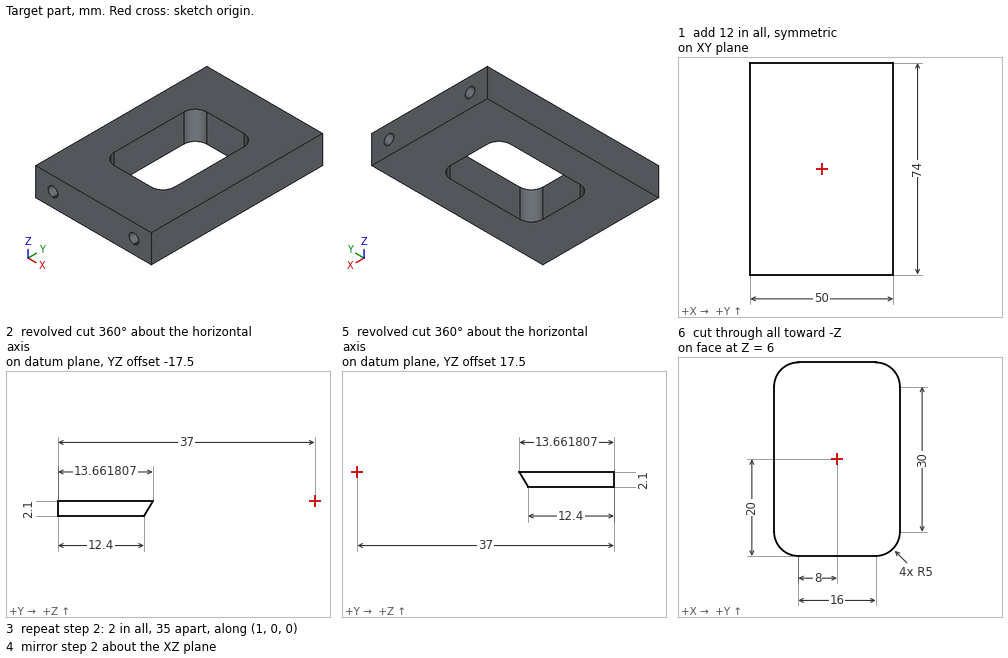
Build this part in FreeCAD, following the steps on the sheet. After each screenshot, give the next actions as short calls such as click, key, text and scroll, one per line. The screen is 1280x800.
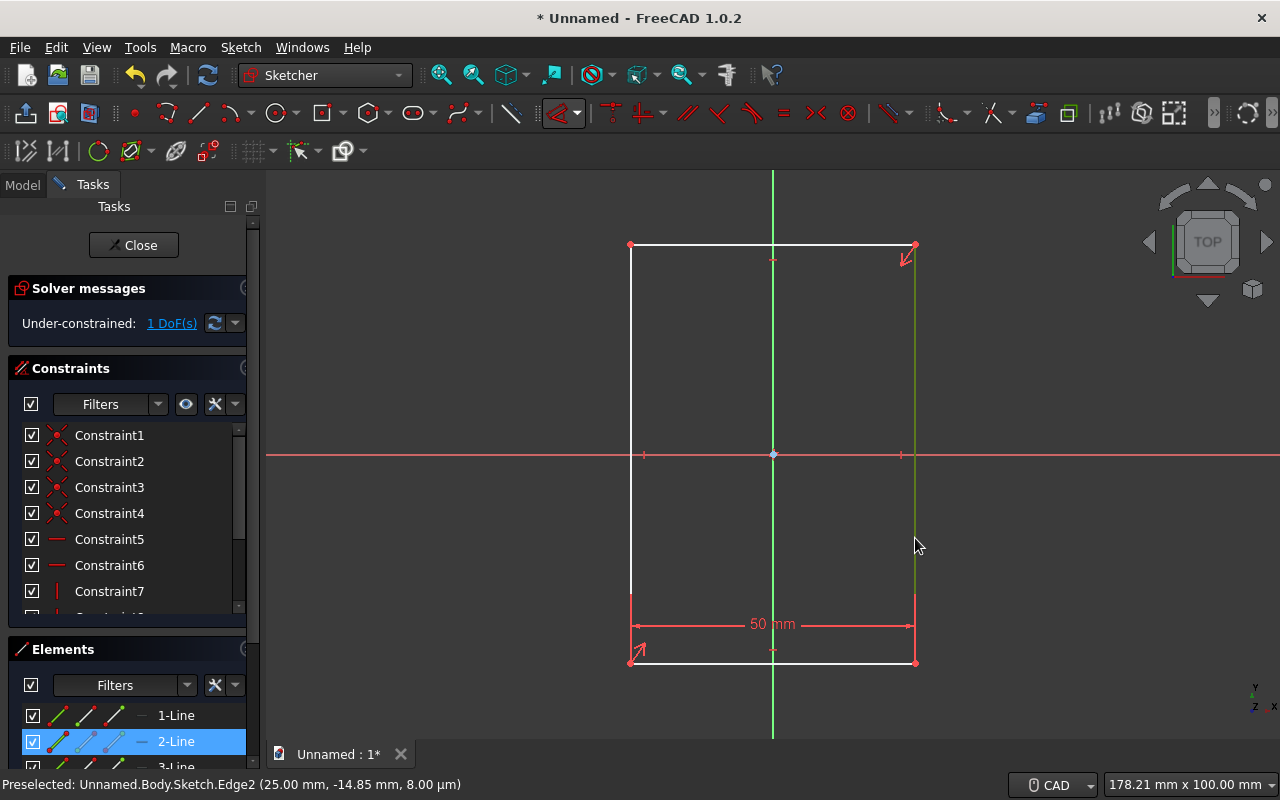
click(580, 114)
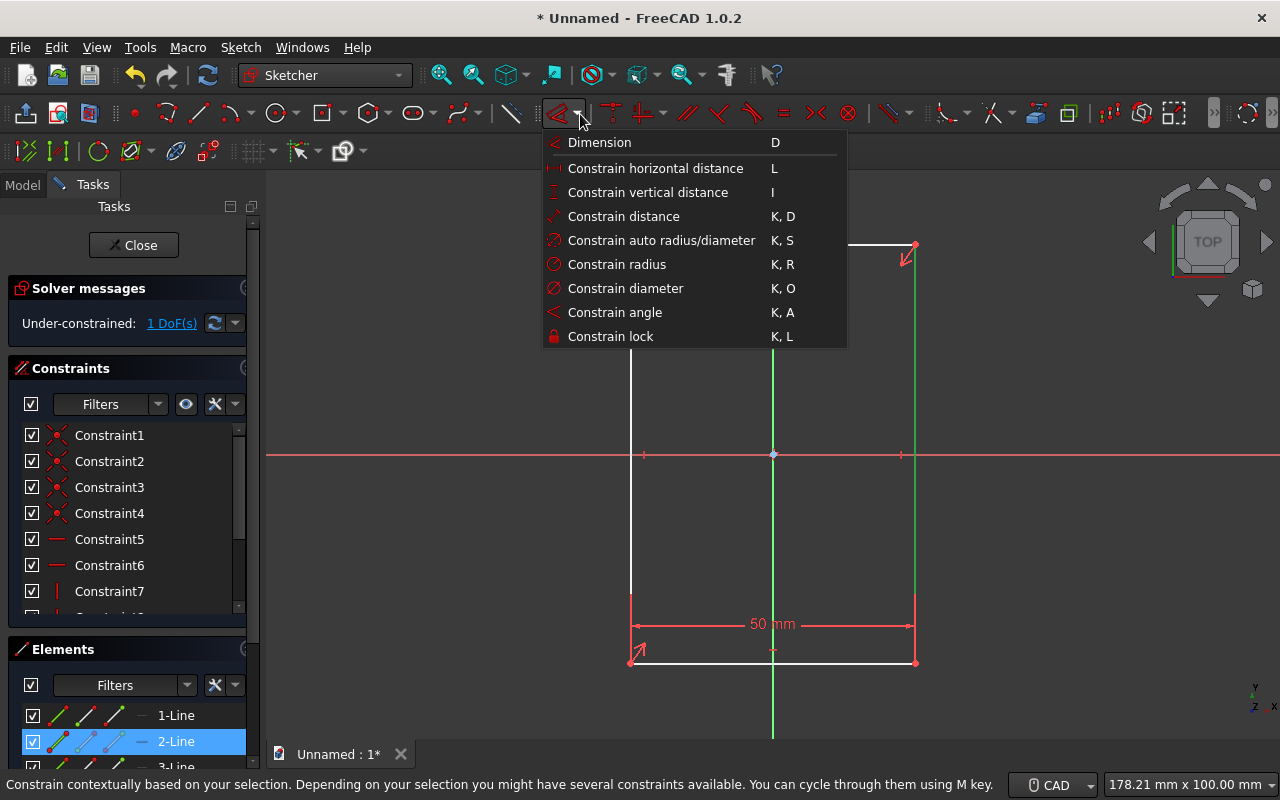
click(695, 192)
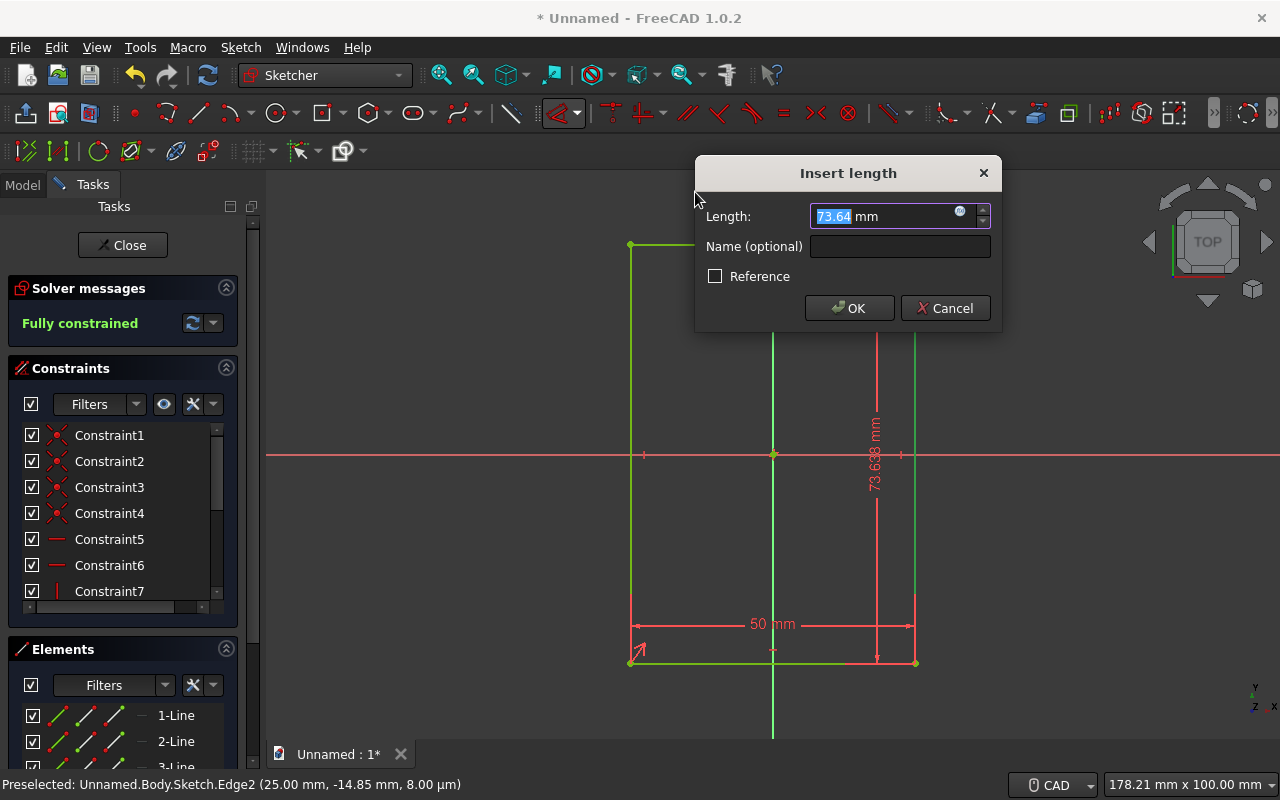
text(74)
key(Return)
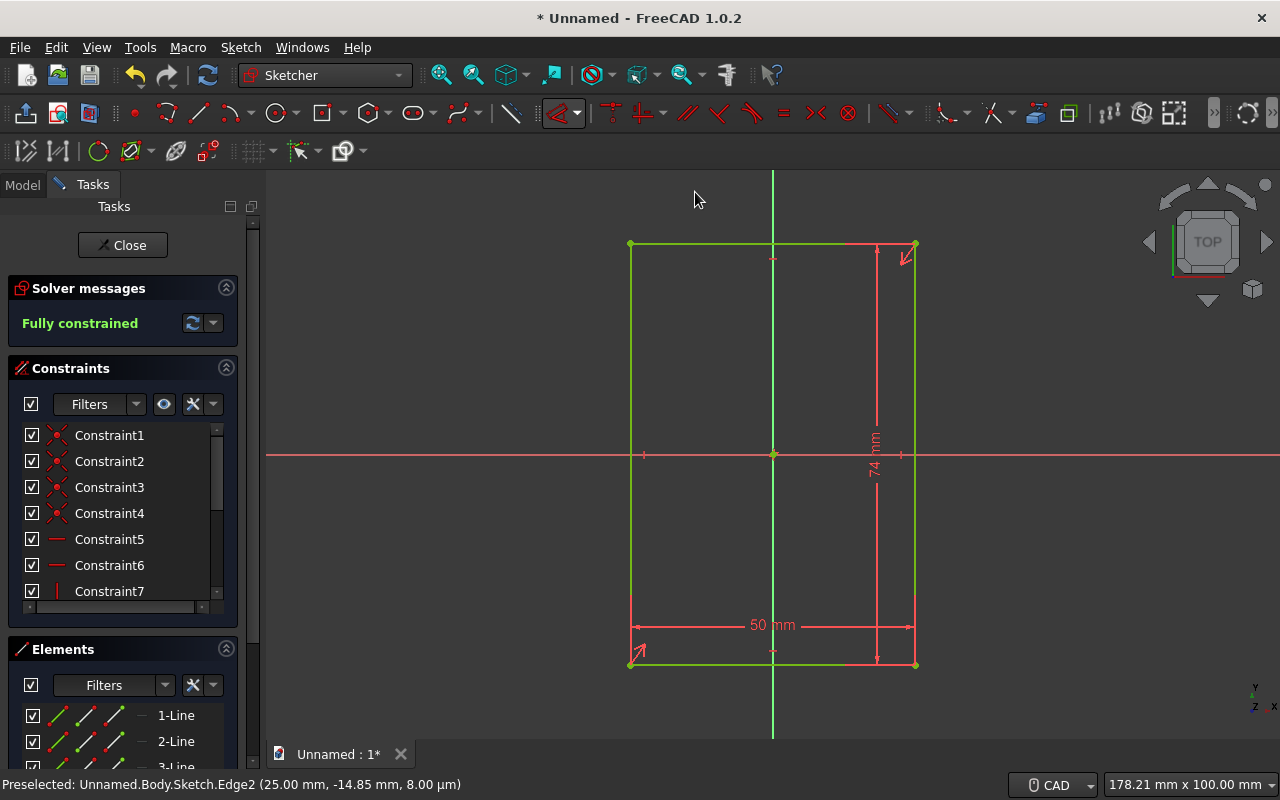
click(123, 245)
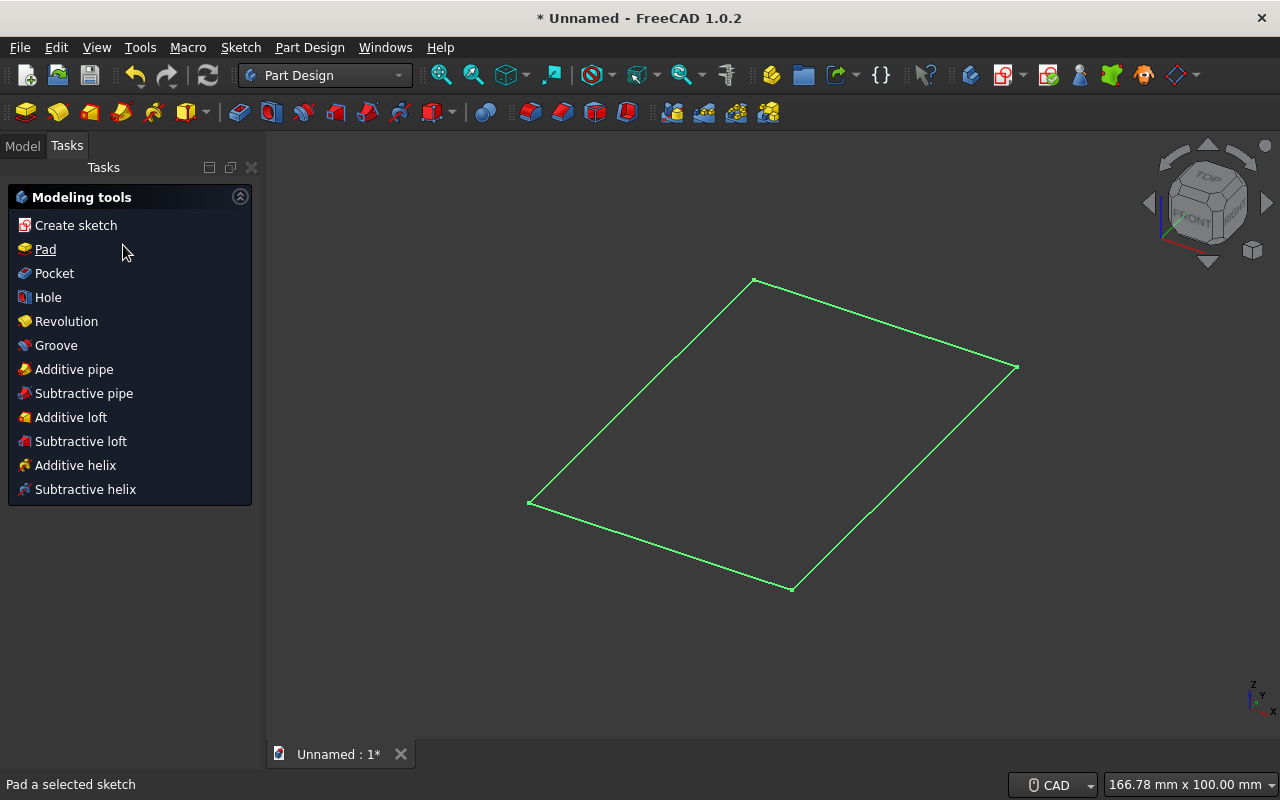
click(26, 112)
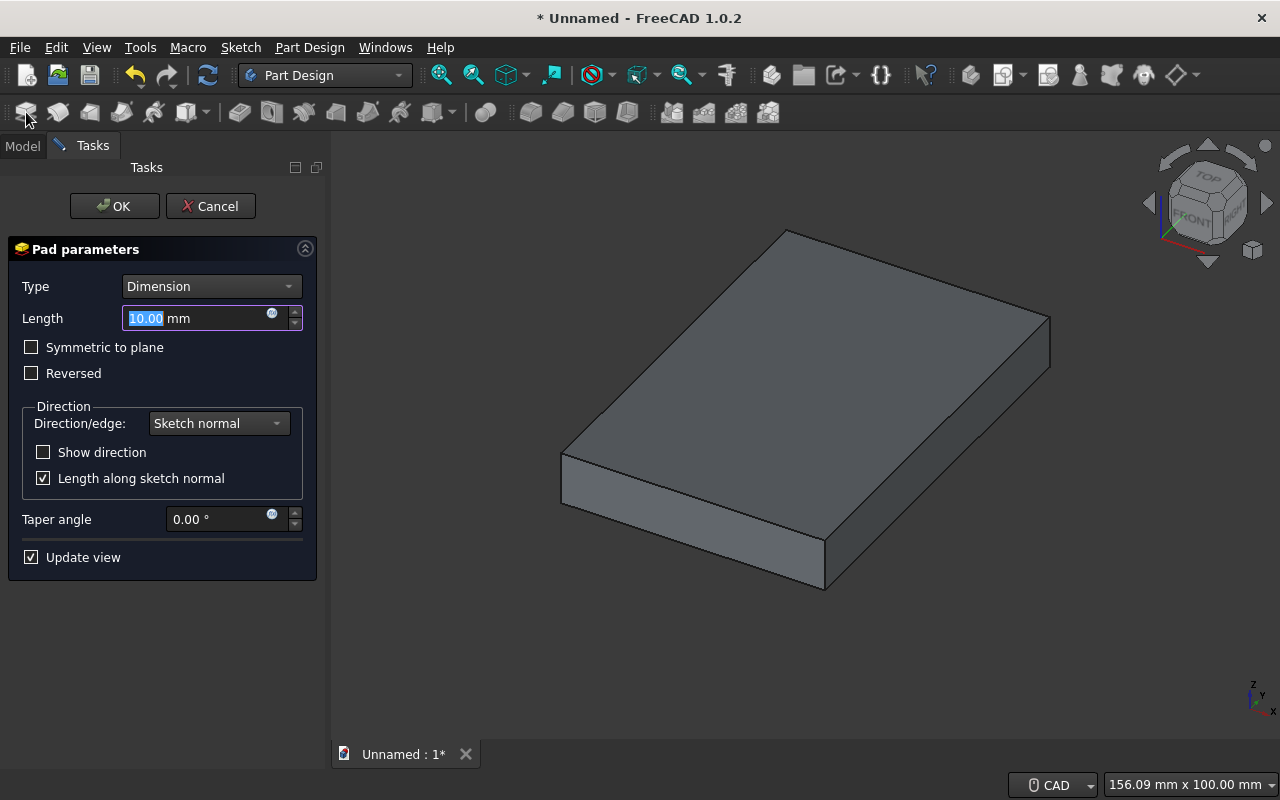
text(12)
key(Tab)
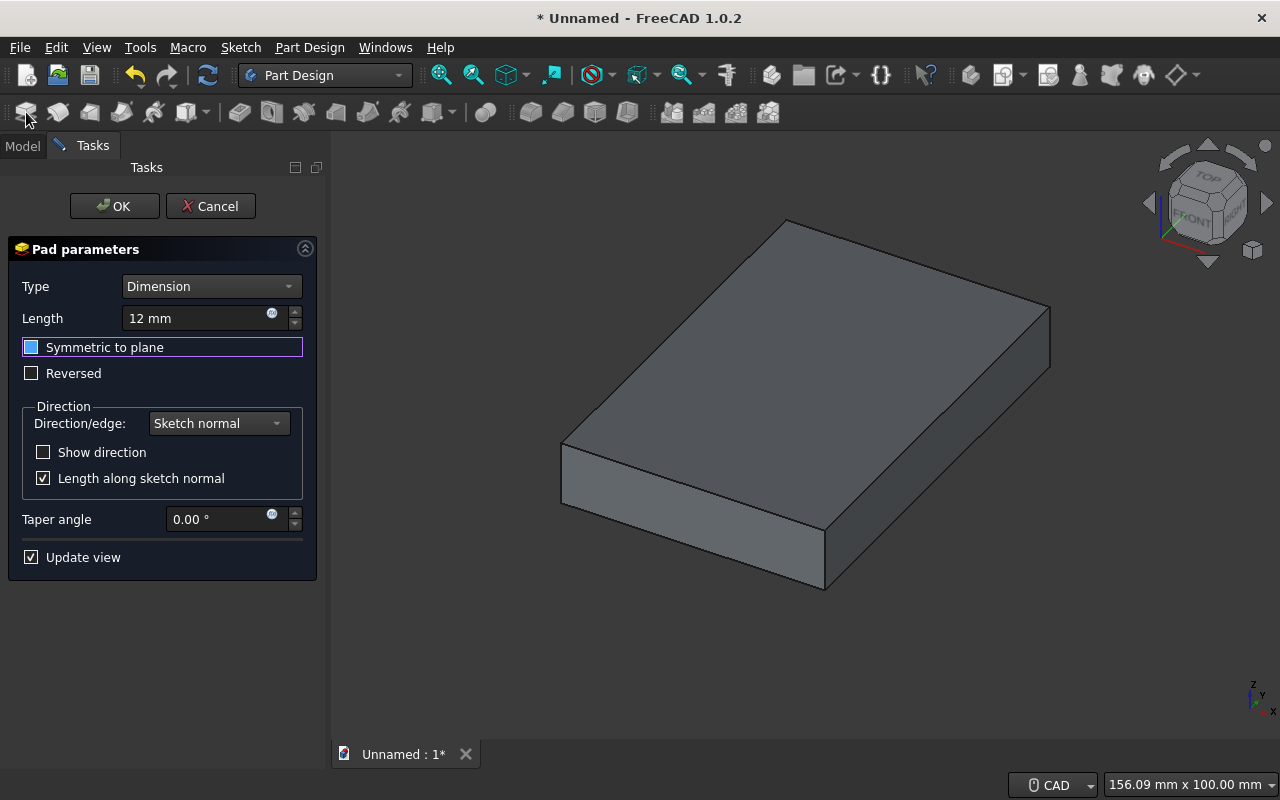
click(30, 347)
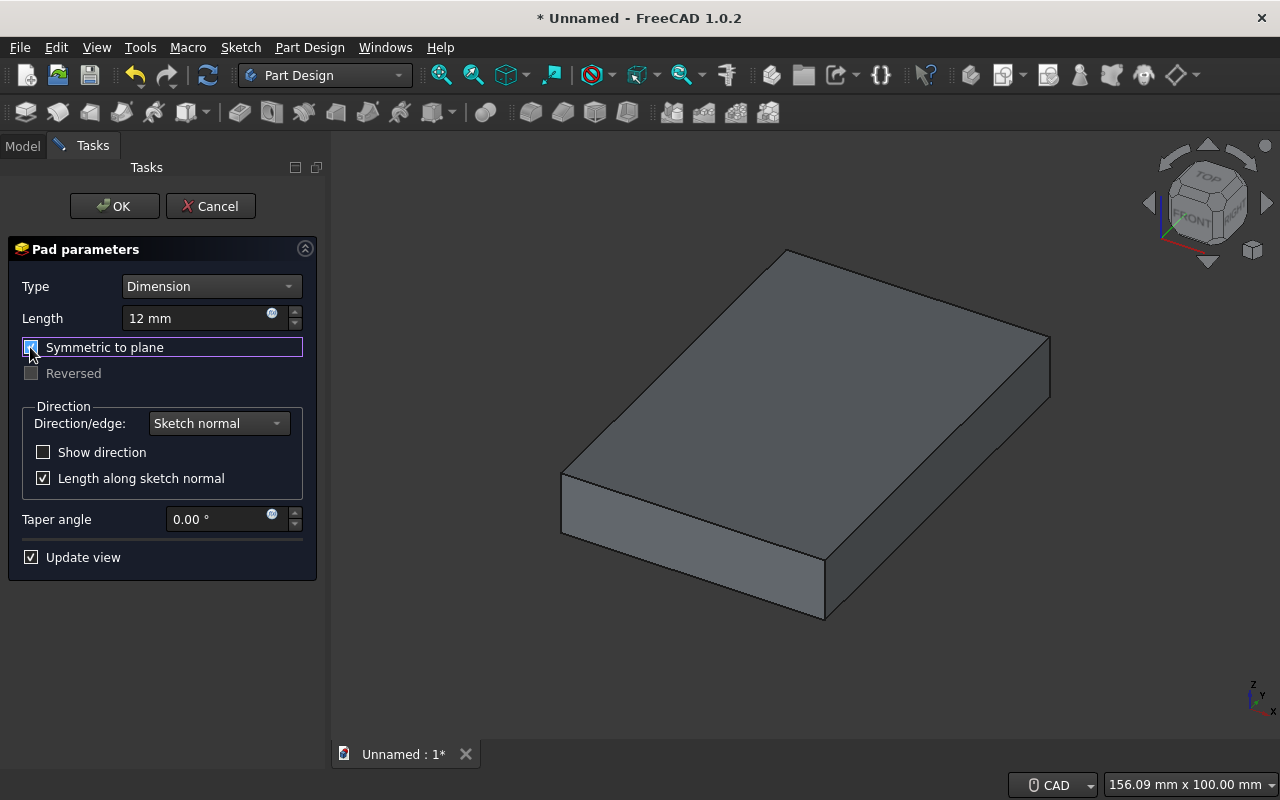
click(115, 206)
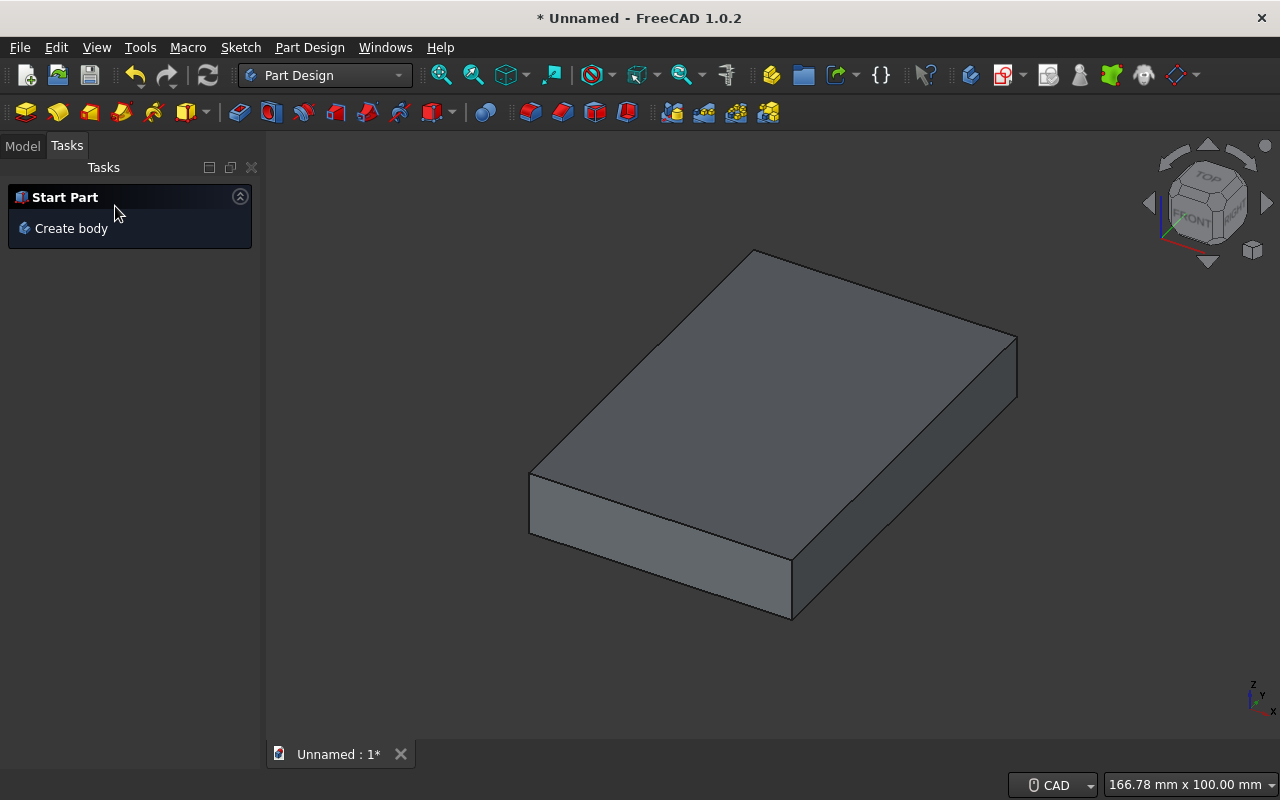
click(23, 145)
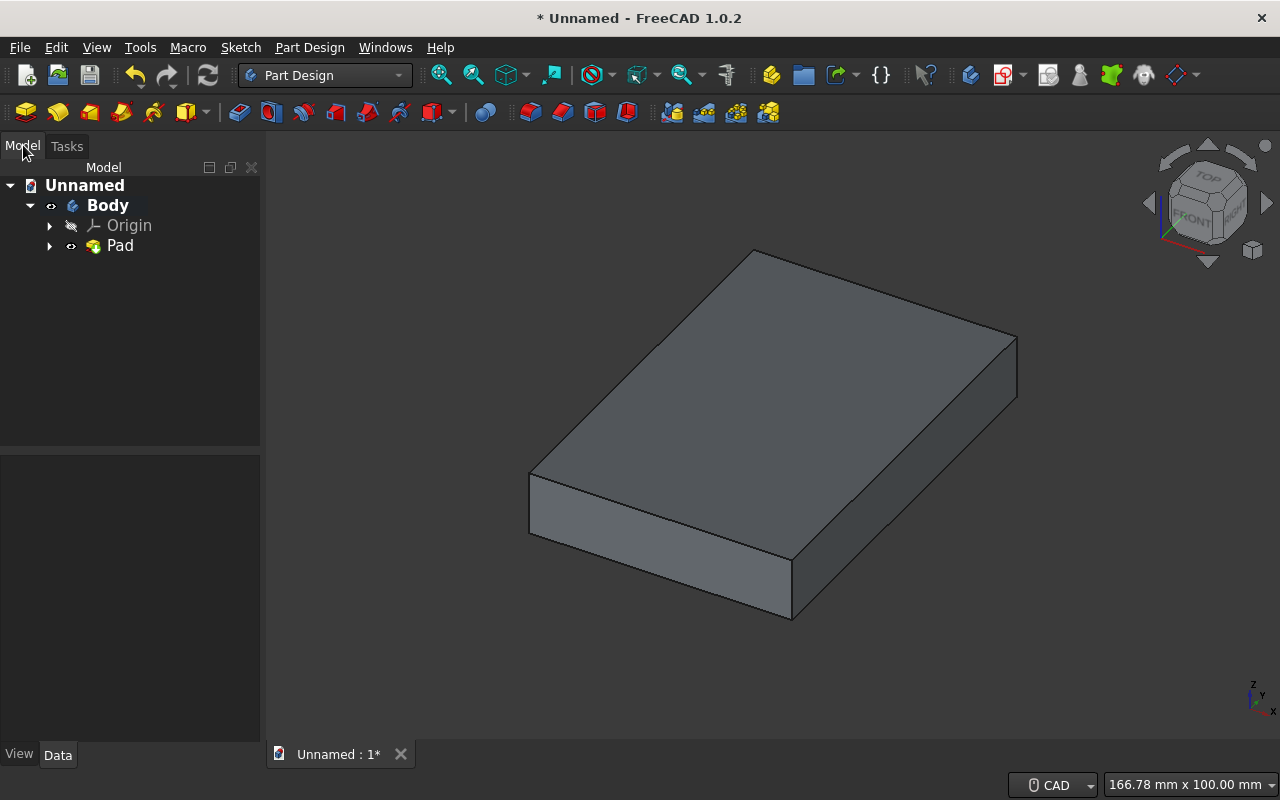
click(50, 226)